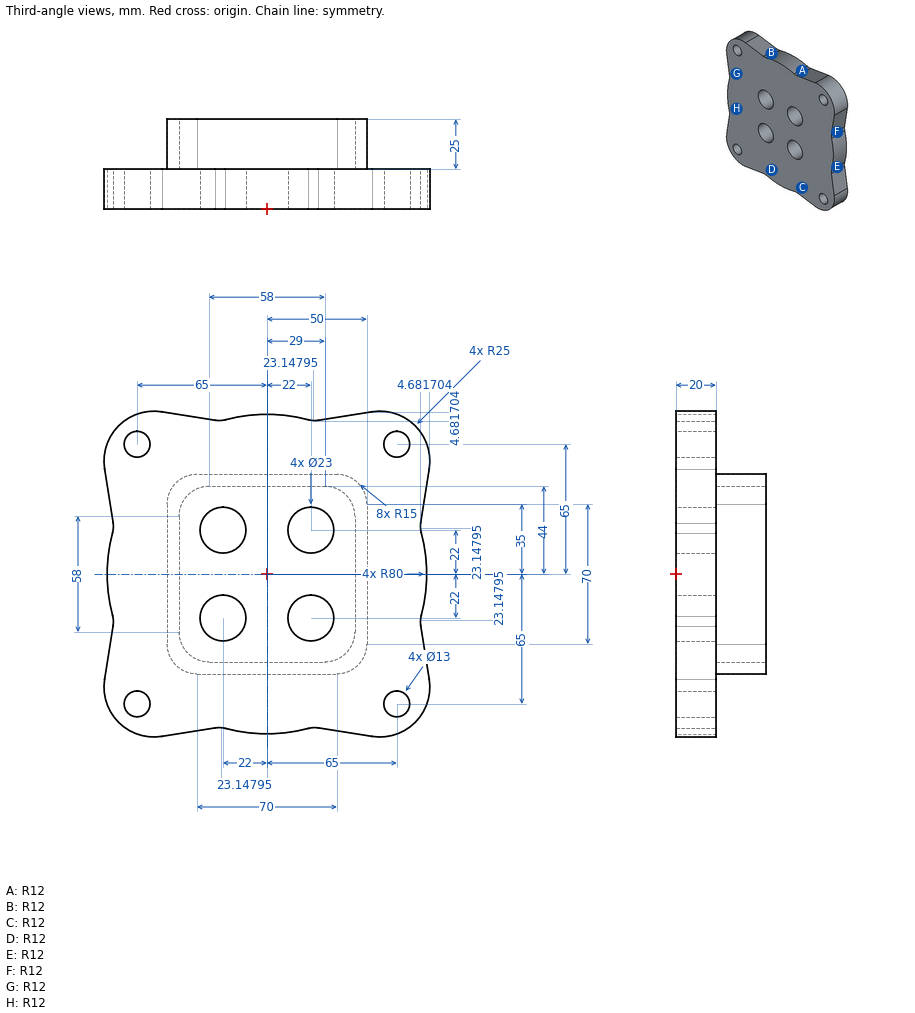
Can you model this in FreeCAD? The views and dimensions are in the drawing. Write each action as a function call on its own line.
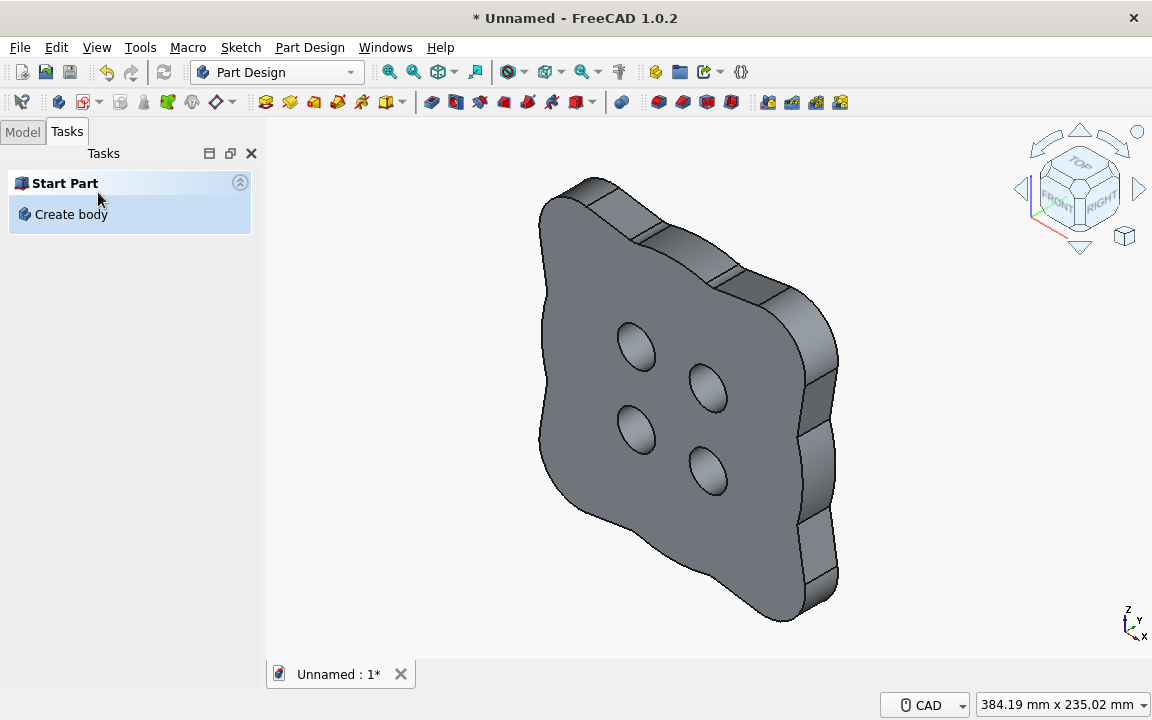
key(2)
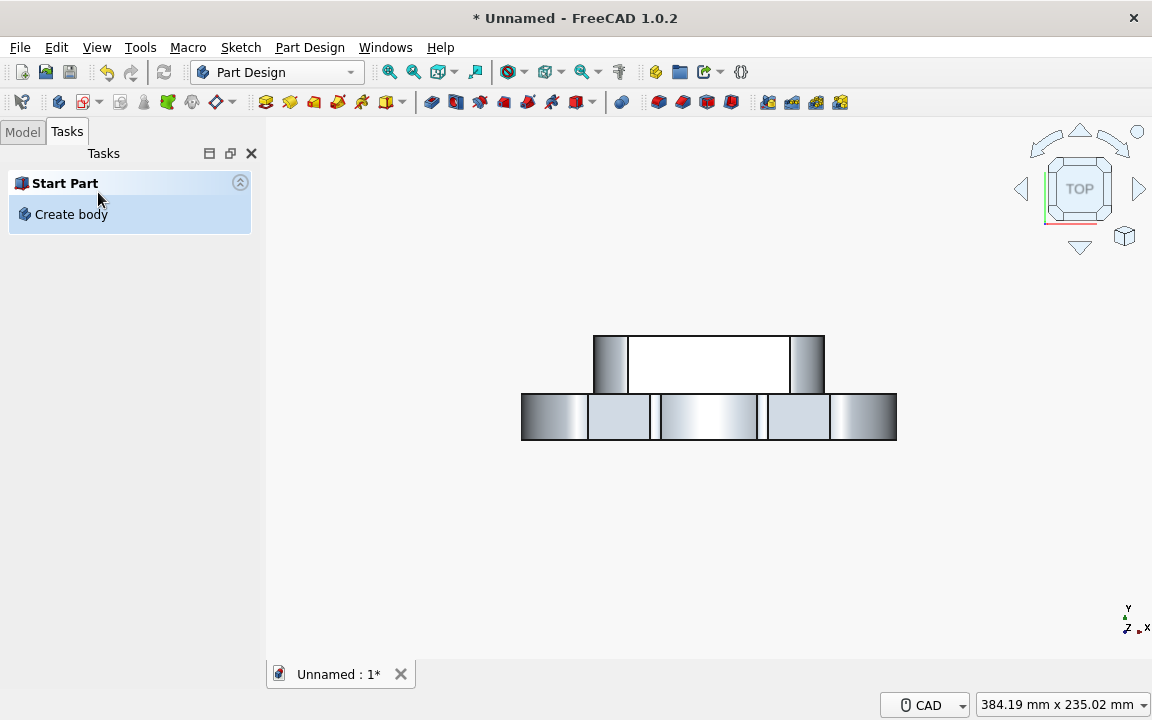
click(390, 72)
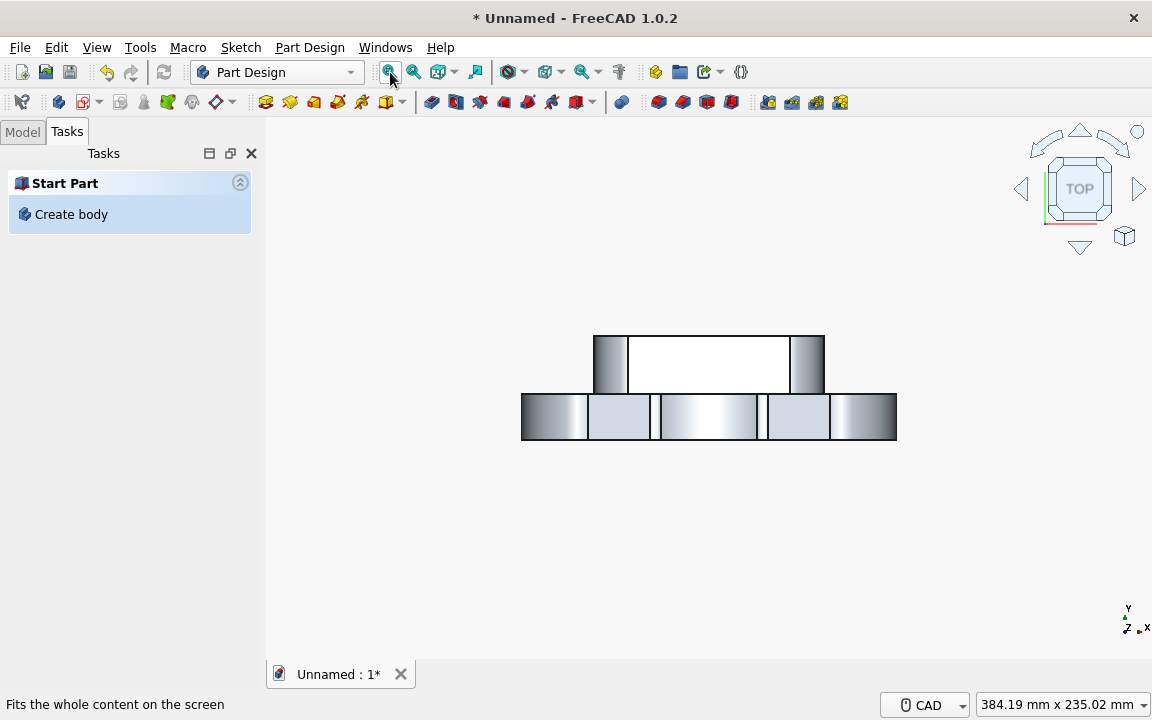
key(0)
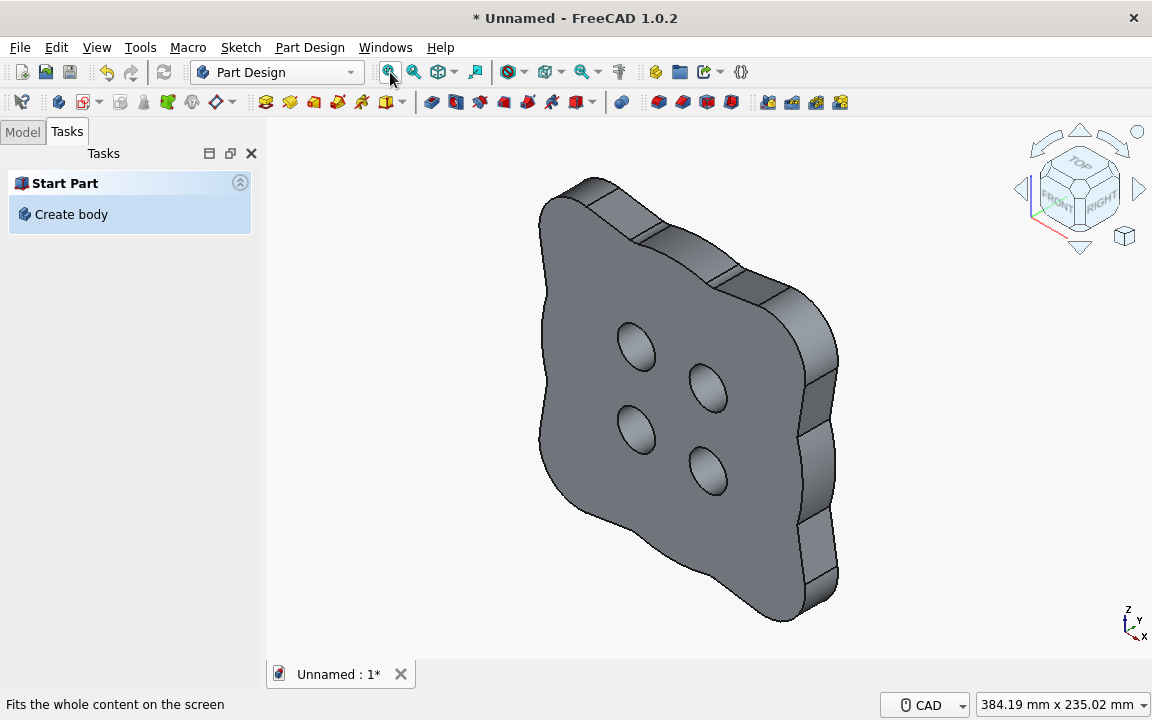
key(1)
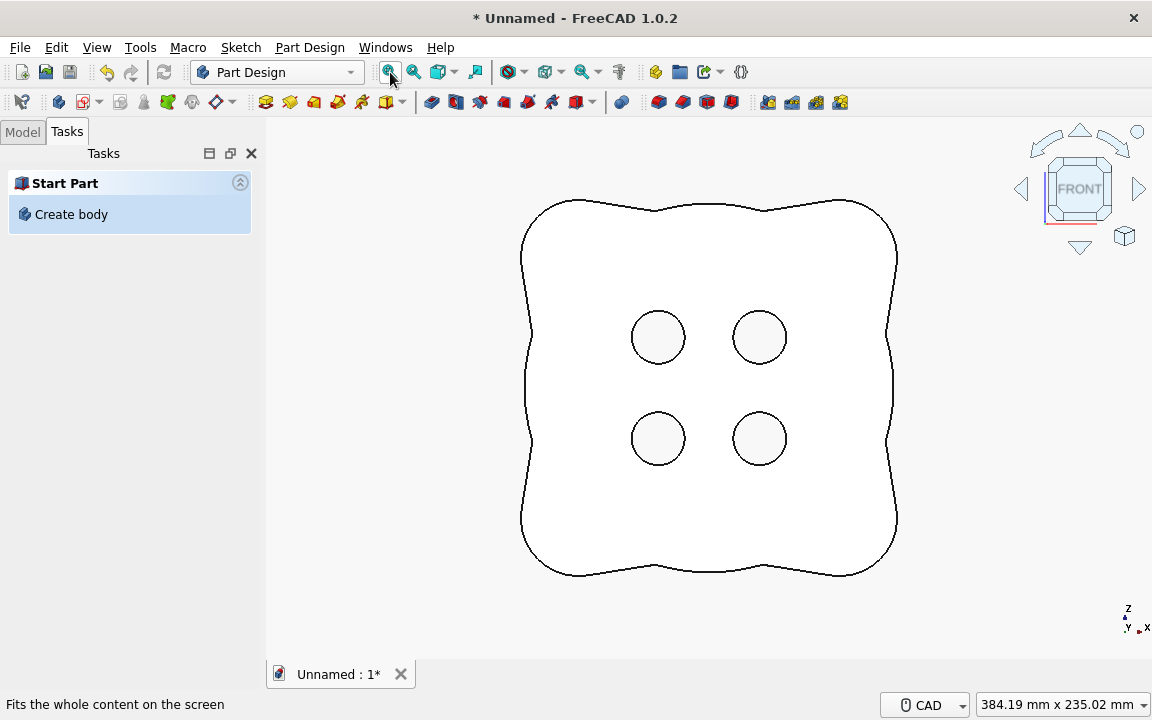
key(3)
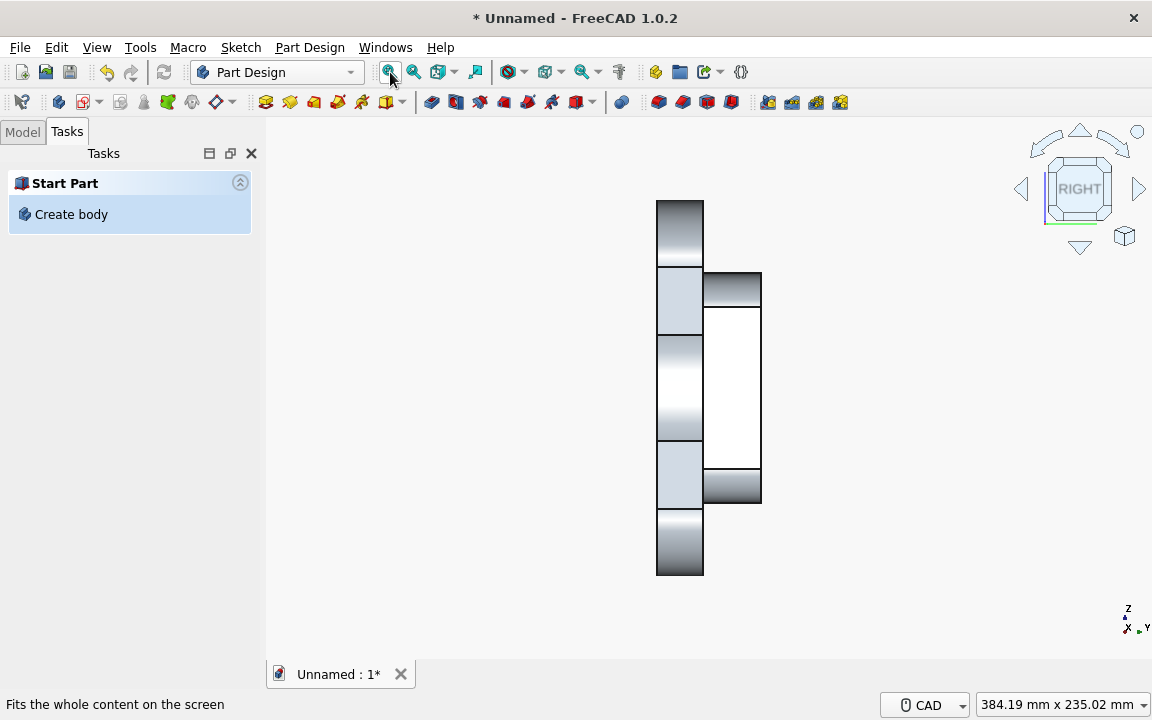
key(5)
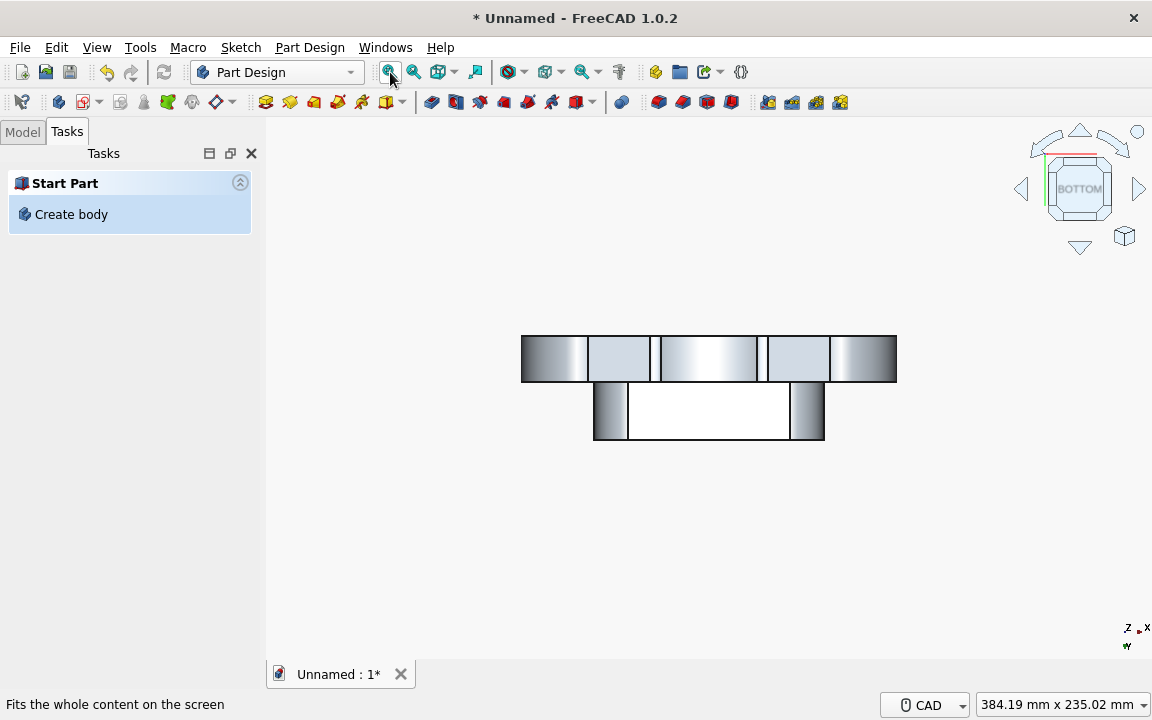
click(390, 72)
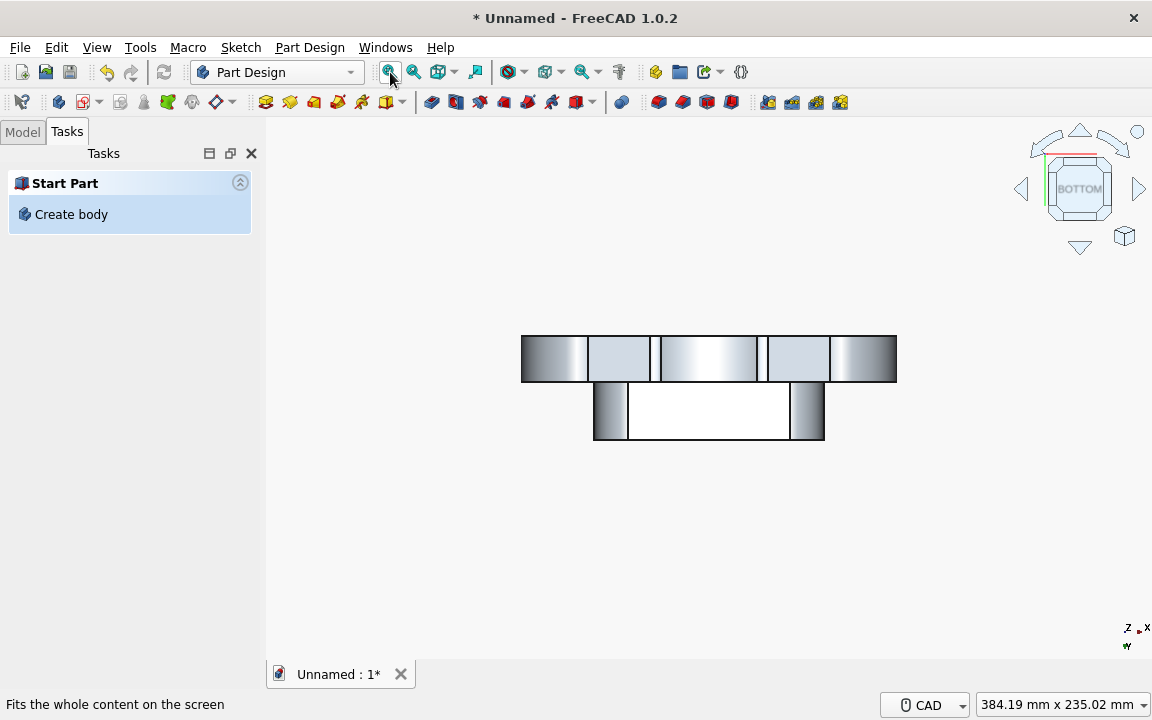
key(4)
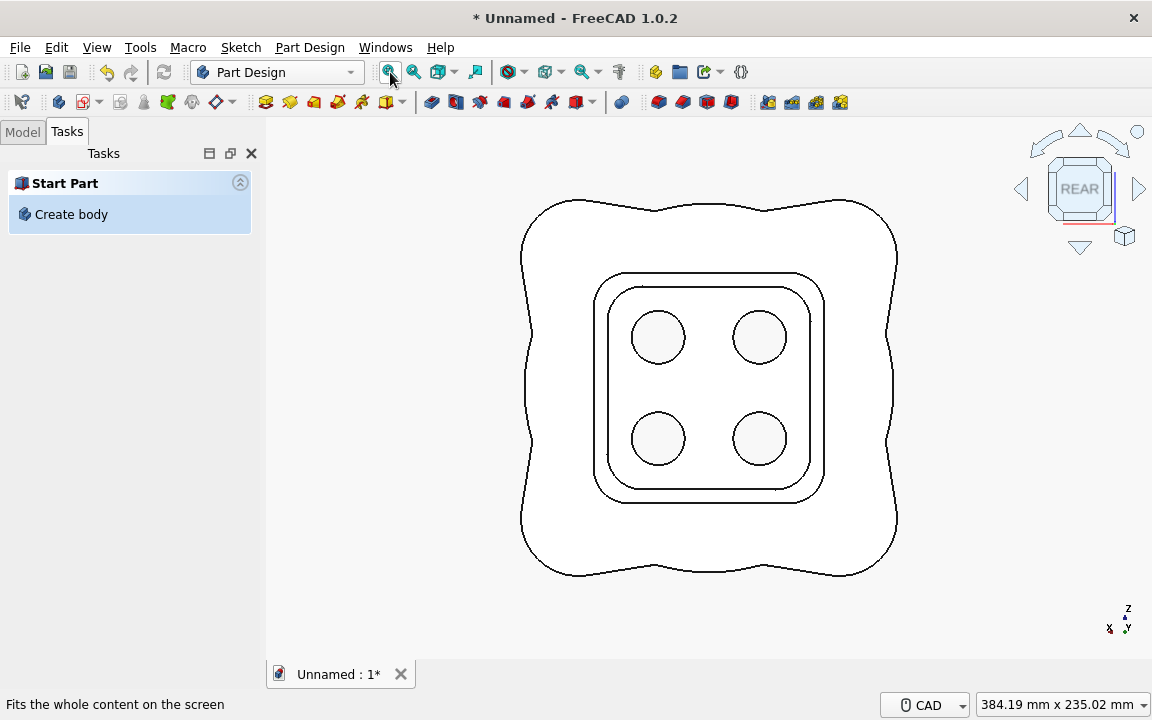
key(6)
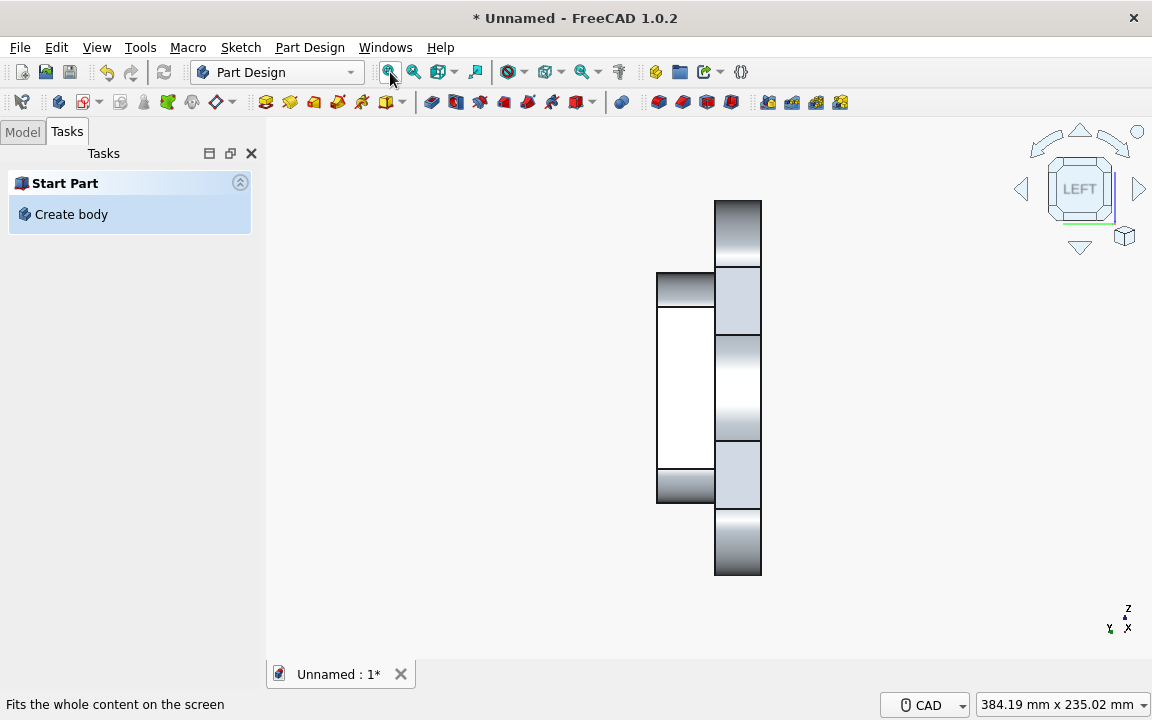
key(v)
key(3)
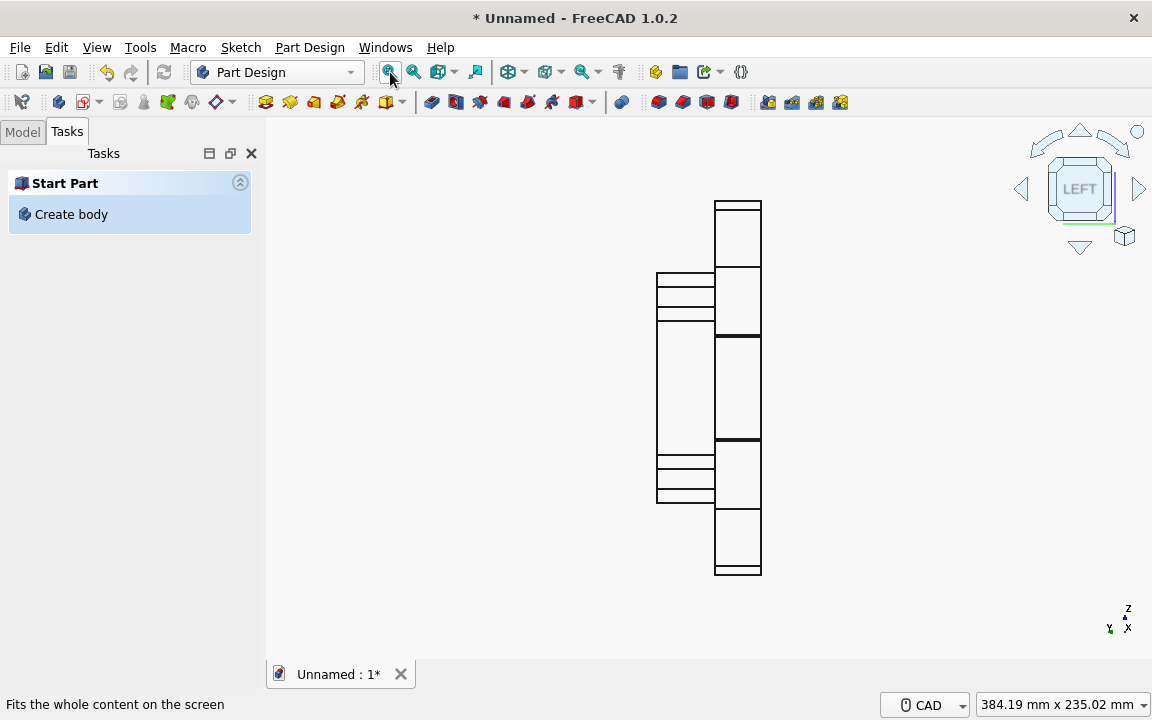
key(0)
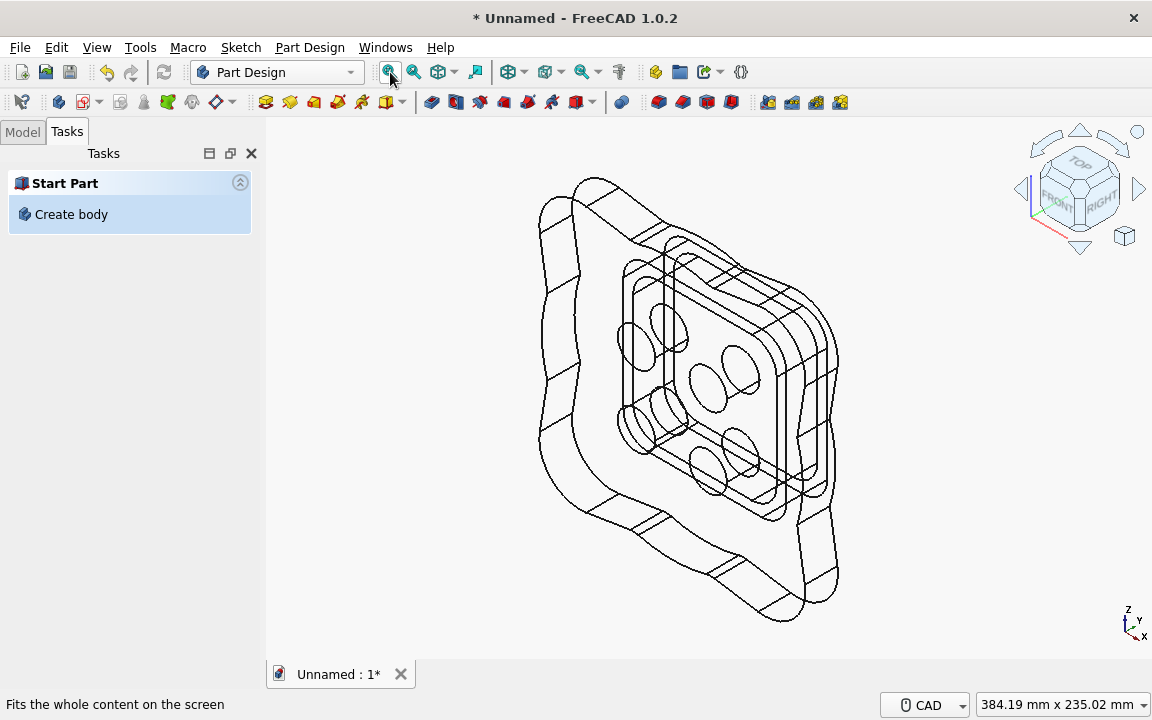
click(813, 514)